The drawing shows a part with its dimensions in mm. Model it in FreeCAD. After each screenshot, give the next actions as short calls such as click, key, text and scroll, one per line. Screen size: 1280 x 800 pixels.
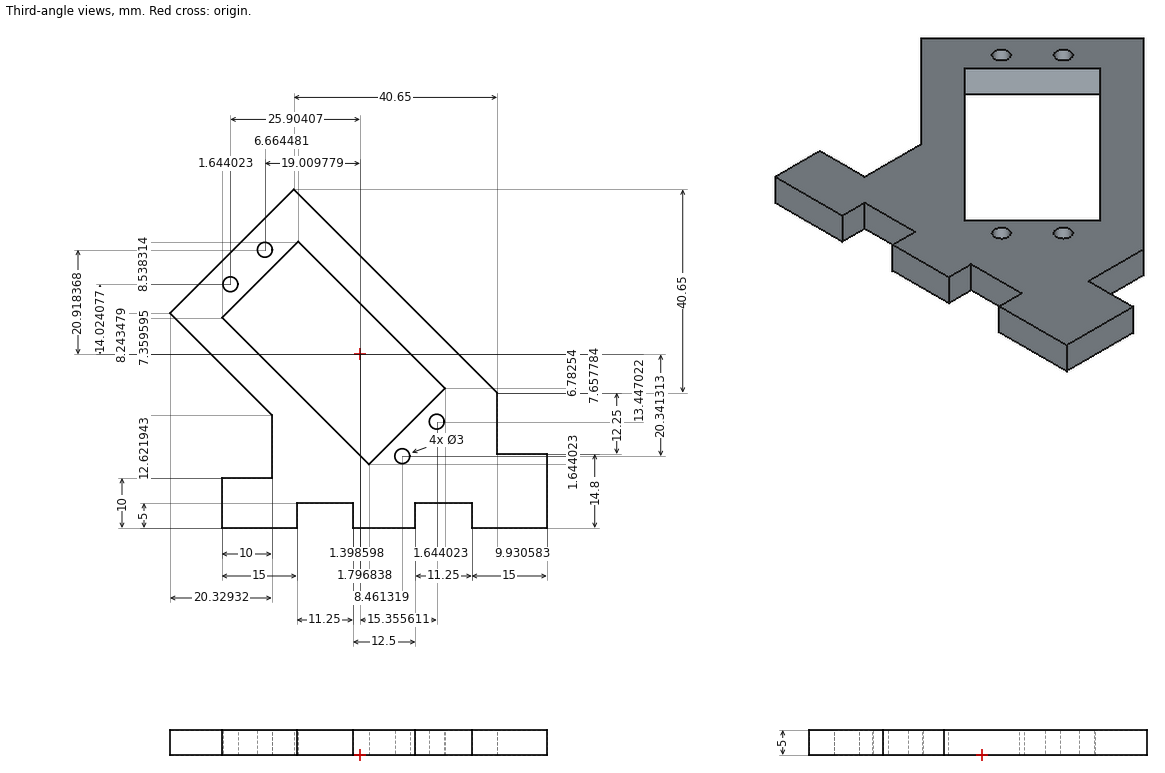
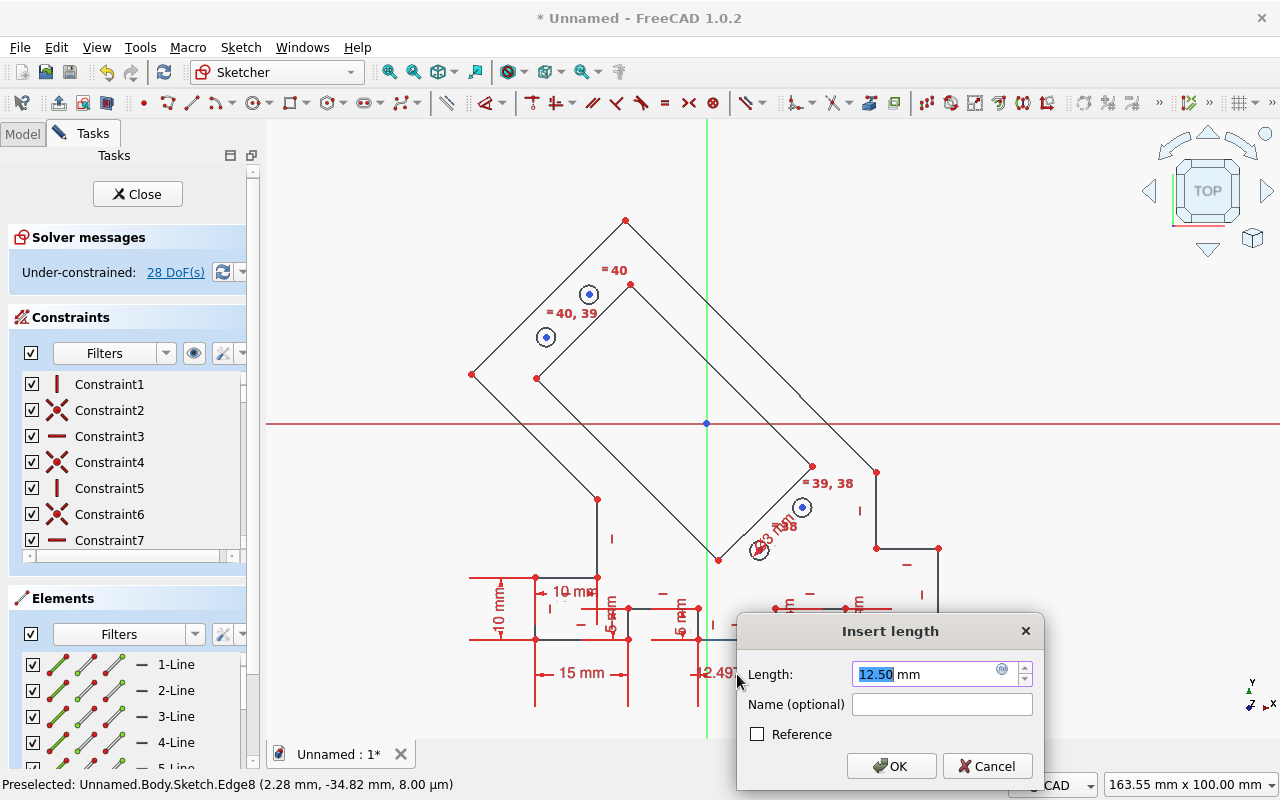
text(12.5)
key(Return)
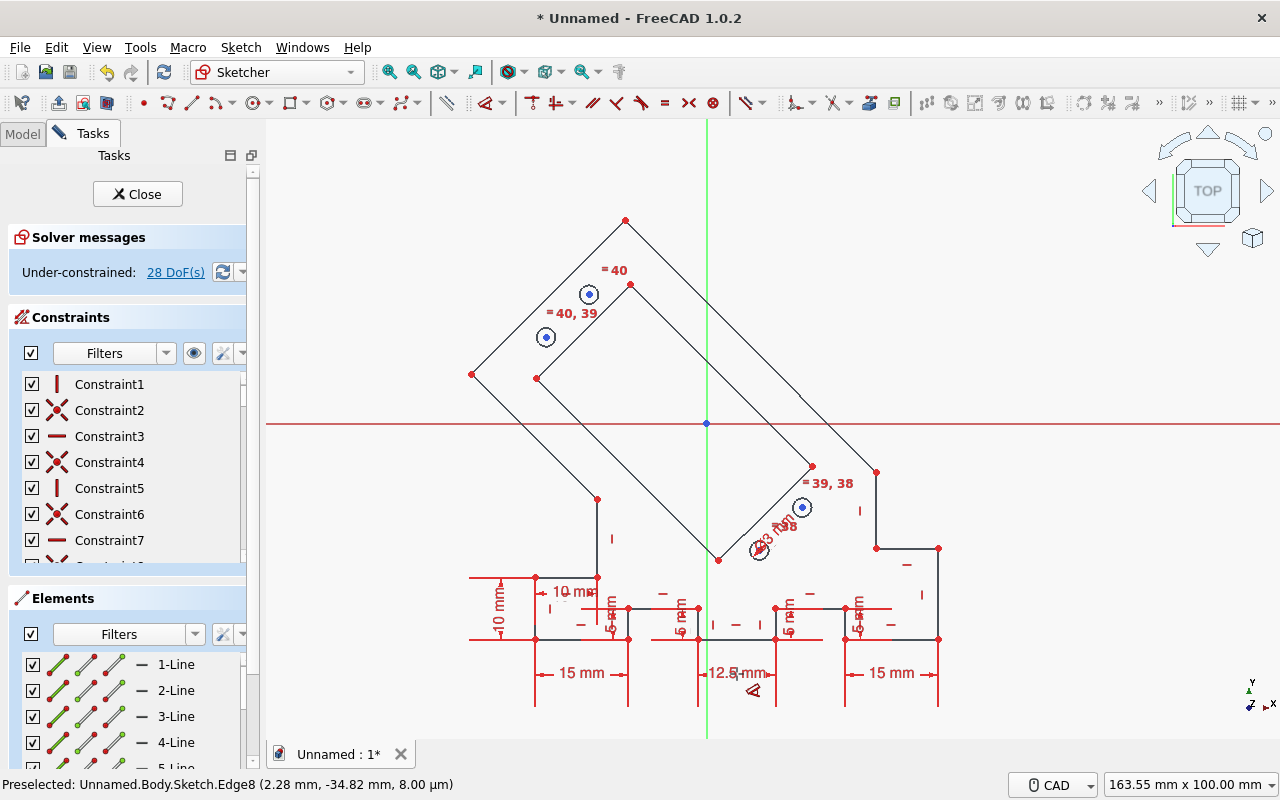
click(938, 612)
click(972, 594)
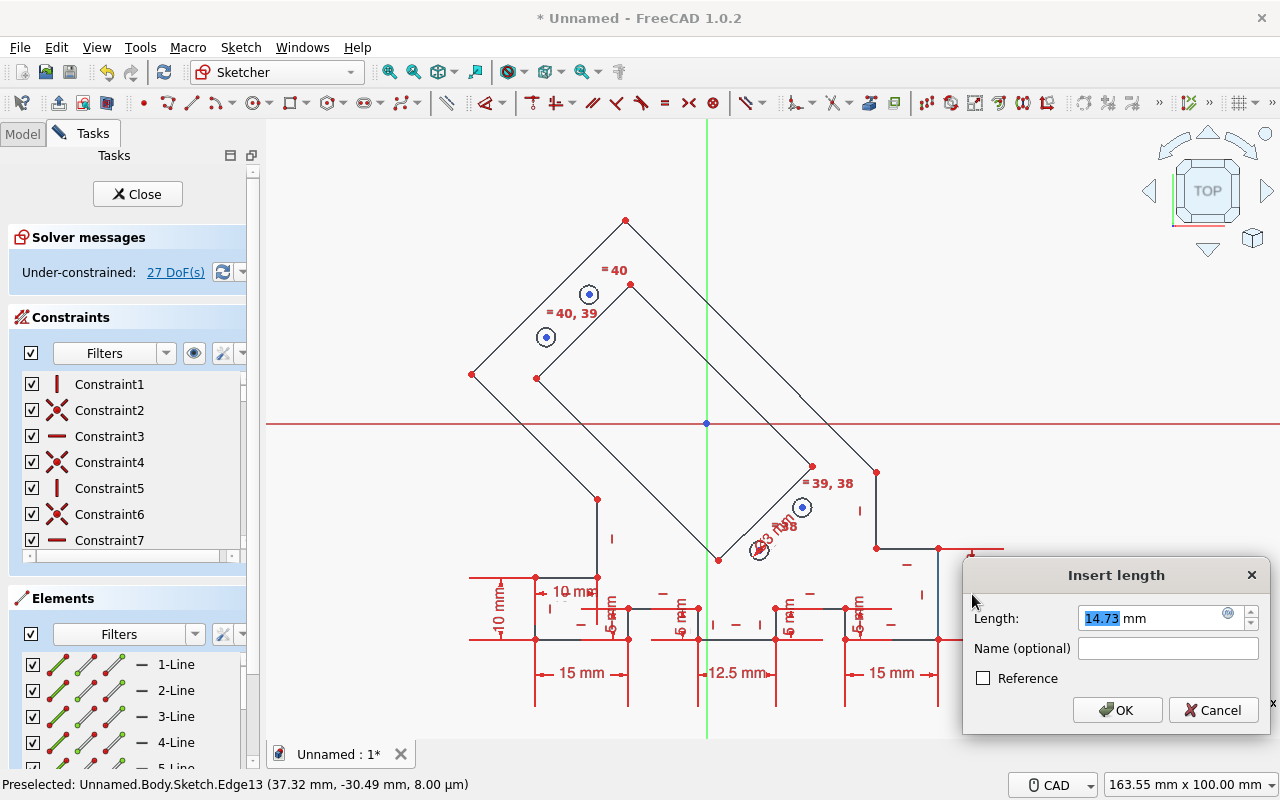
text(14.8)
key(Return)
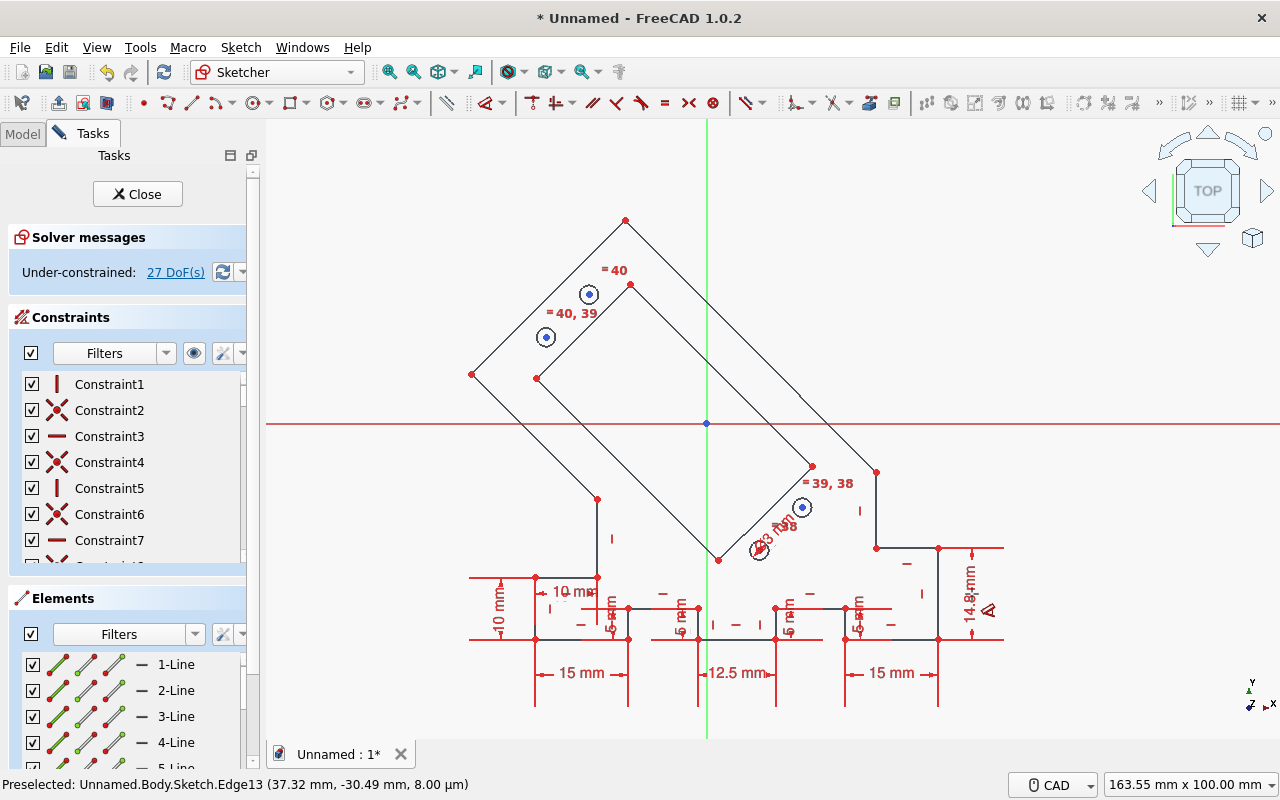
click(649, 609)
click(663, 643)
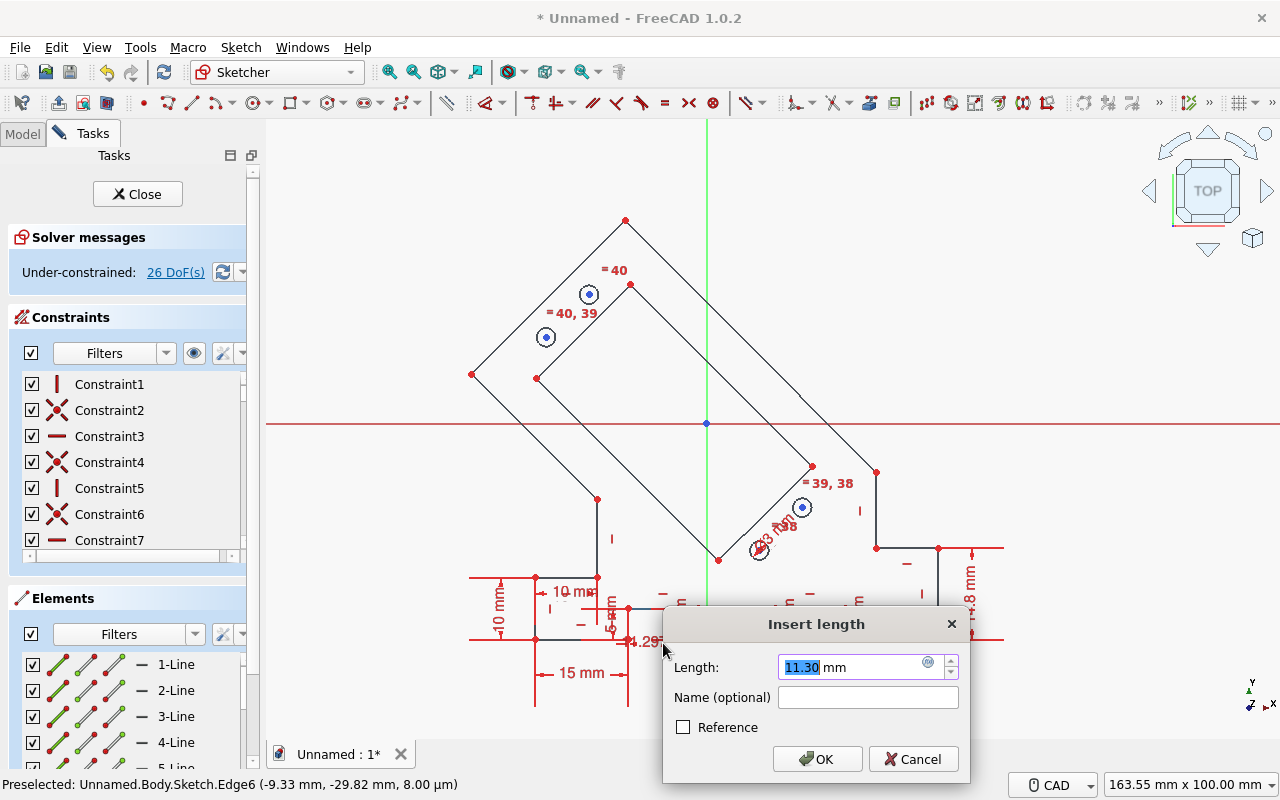
text(11.25)
key(Return)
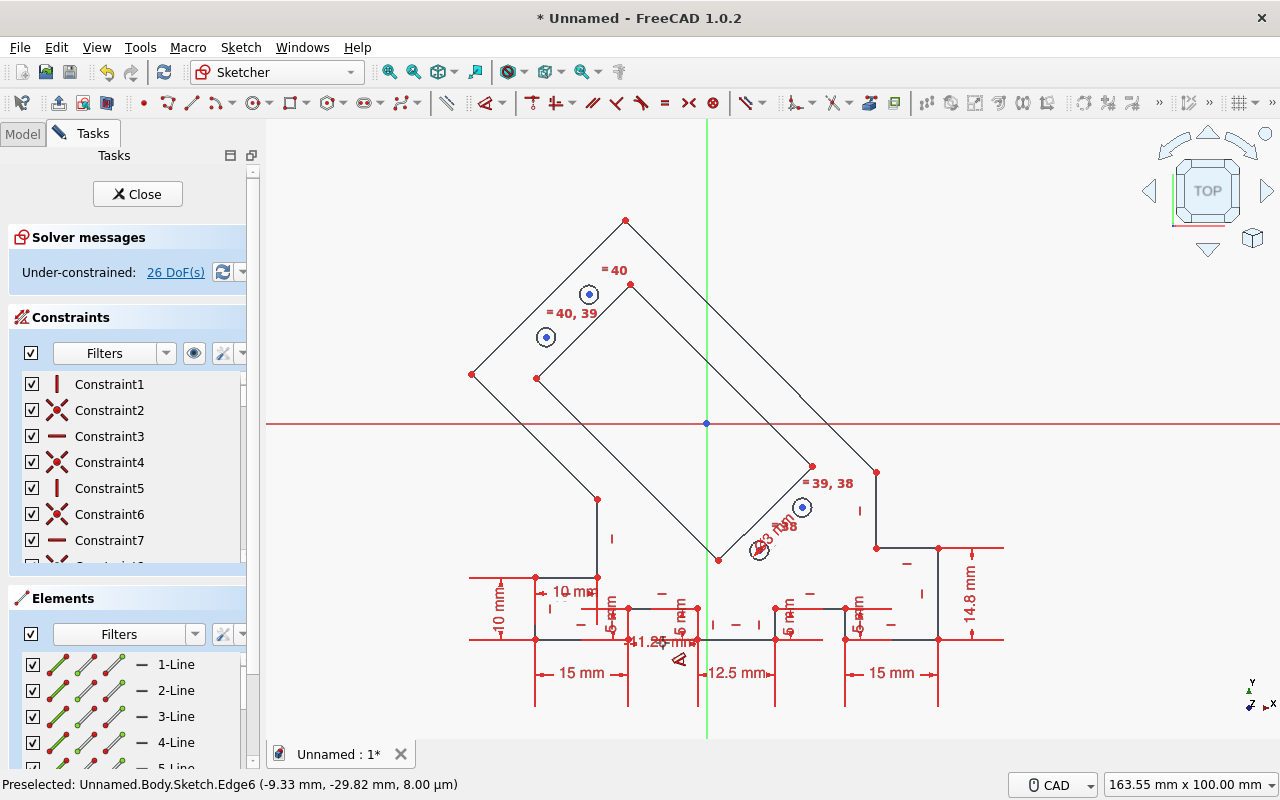
click(796, 609)
click(810, 643)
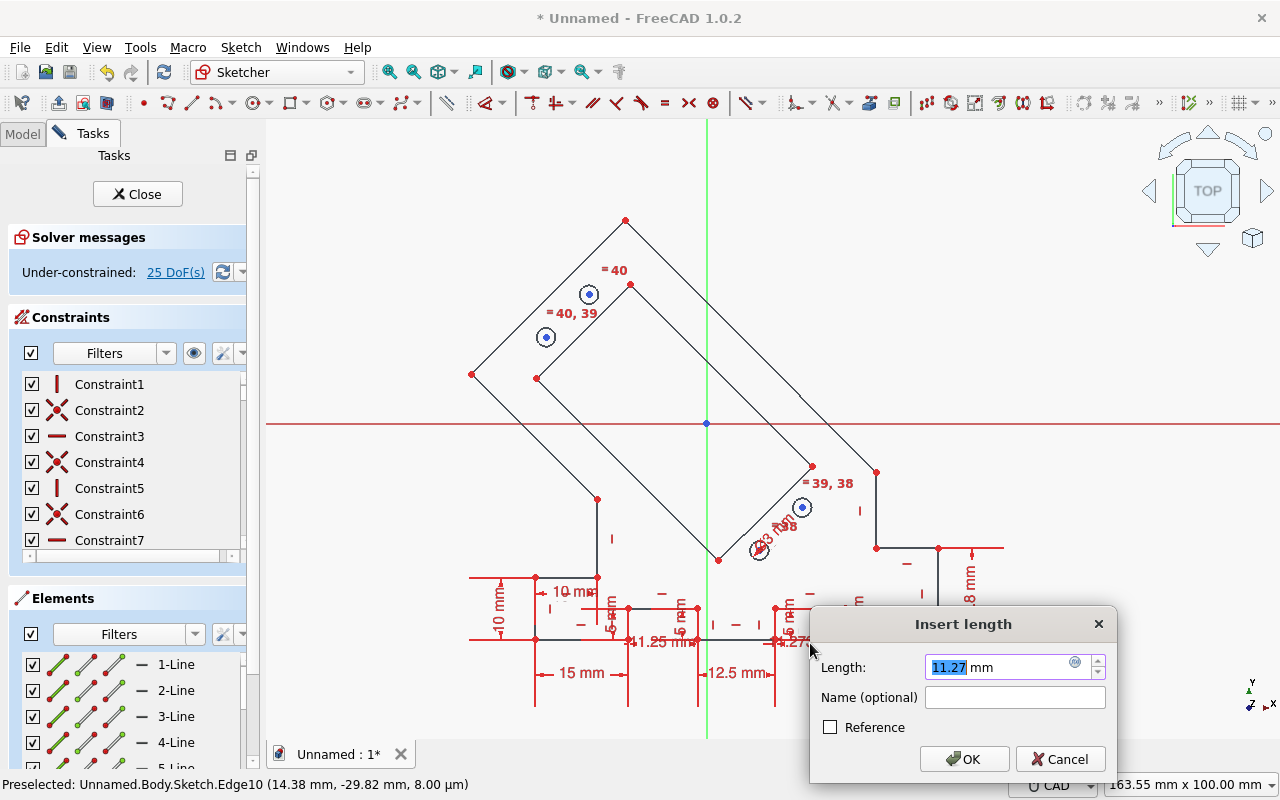
text(11.25)
key(Return)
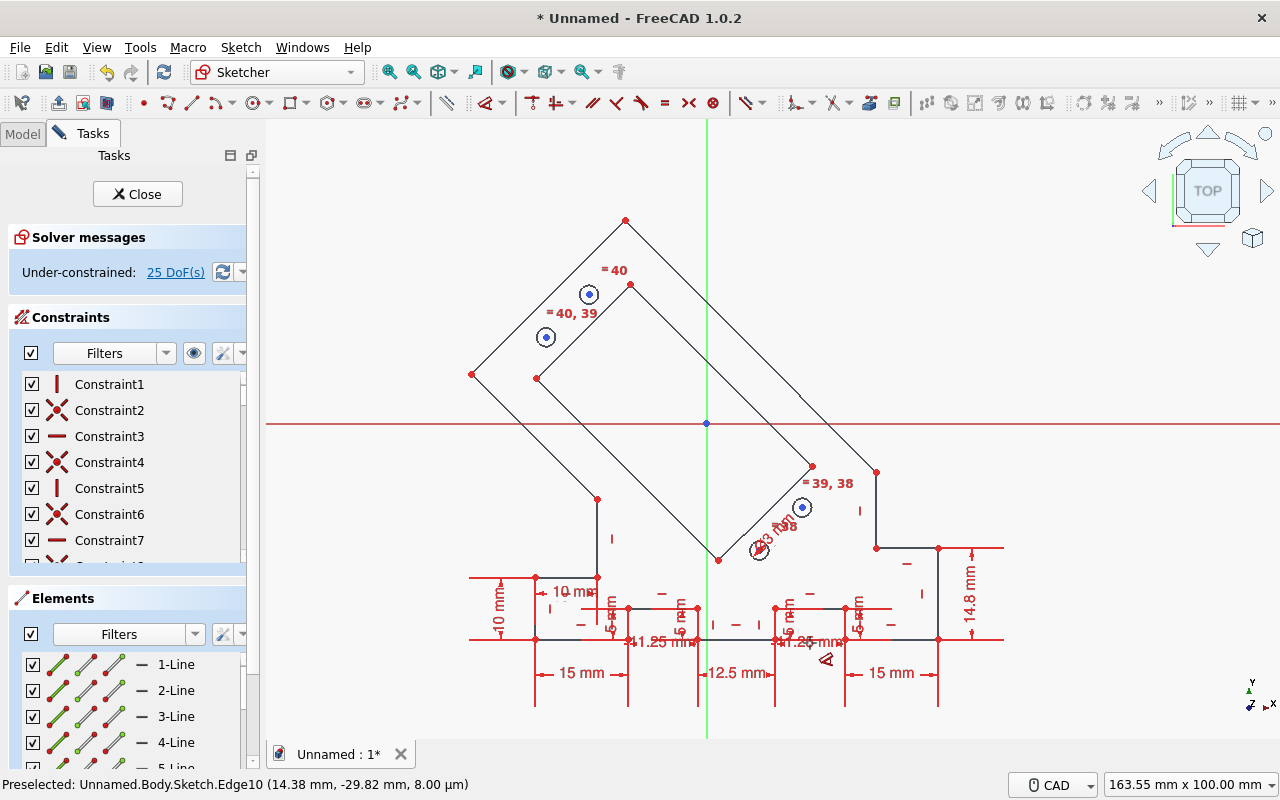
click(876, 525)
click(910, 510)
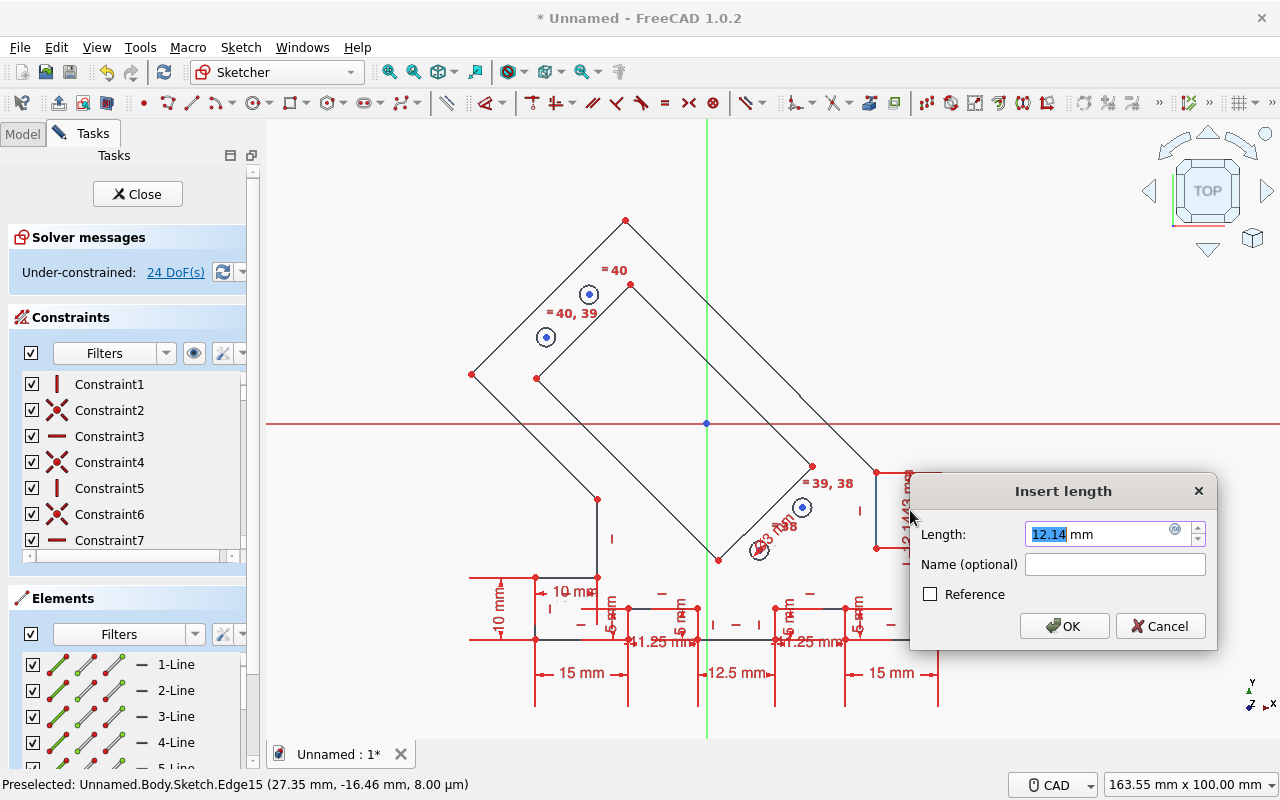
text(12.25)
key(Return)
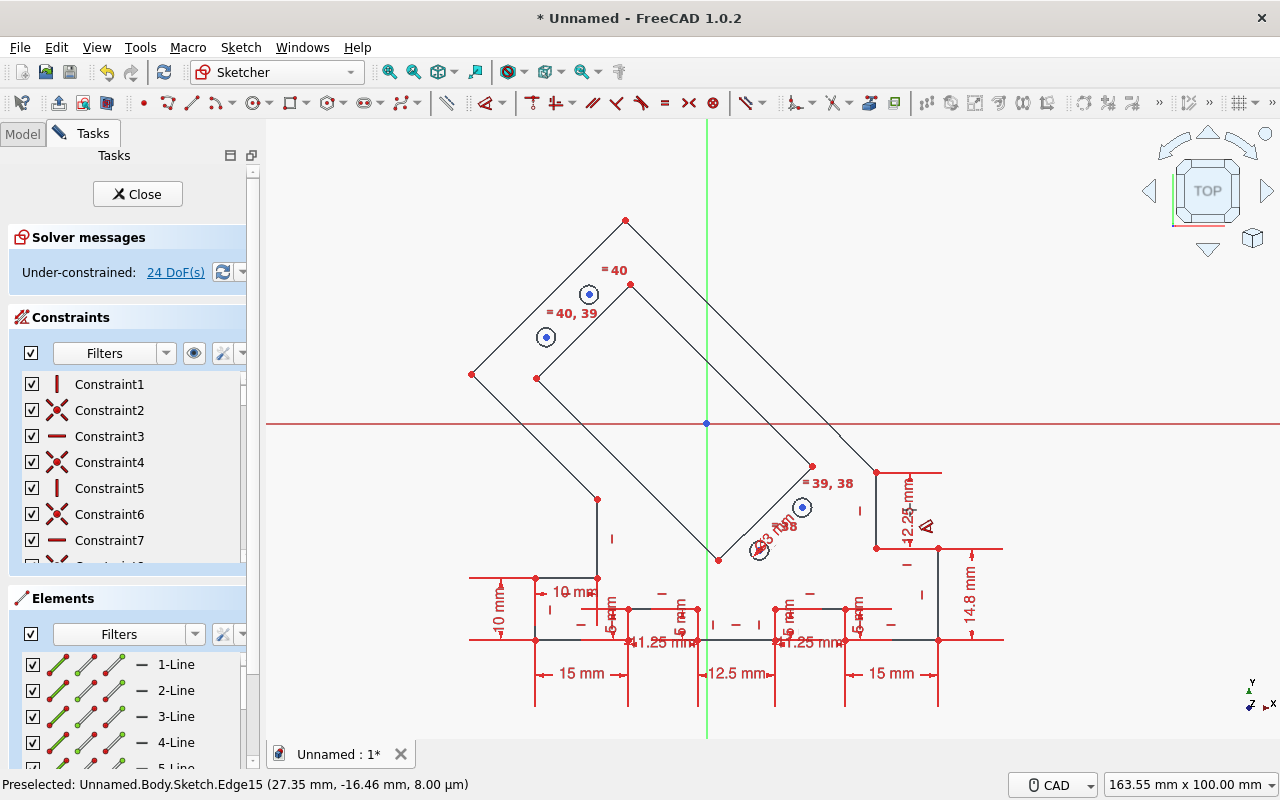
click(801, 397)
click(751, 187)